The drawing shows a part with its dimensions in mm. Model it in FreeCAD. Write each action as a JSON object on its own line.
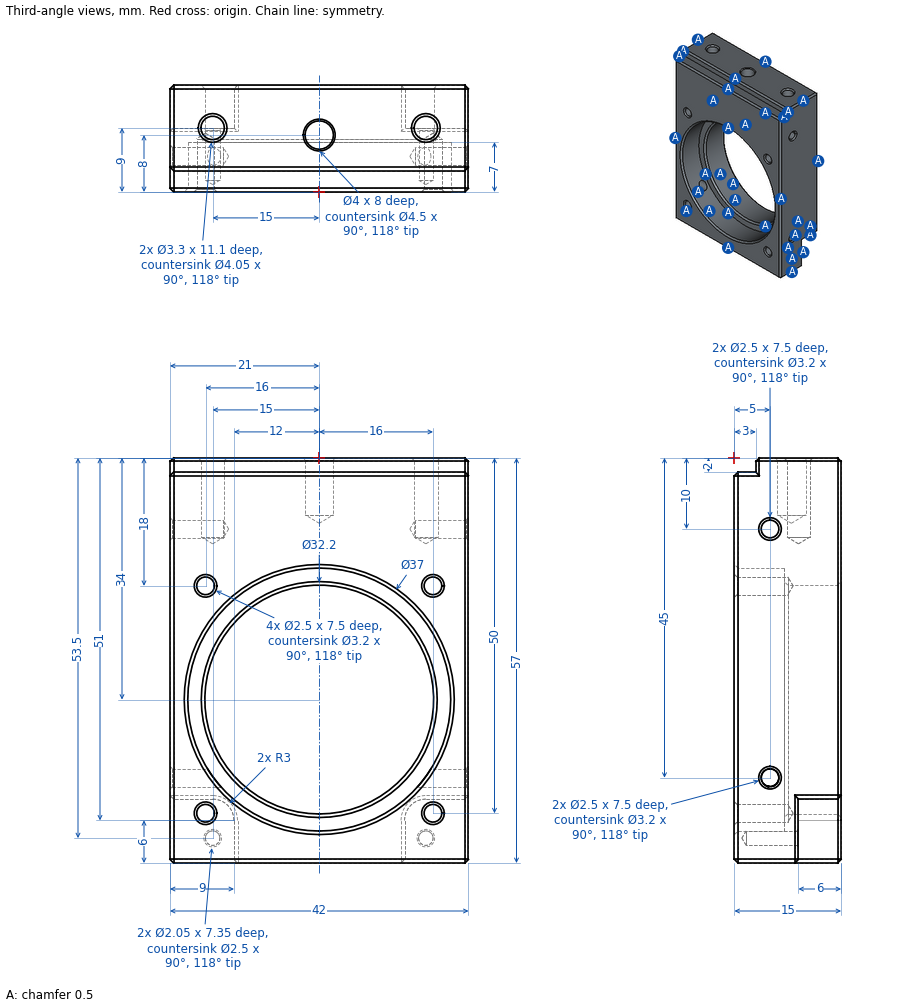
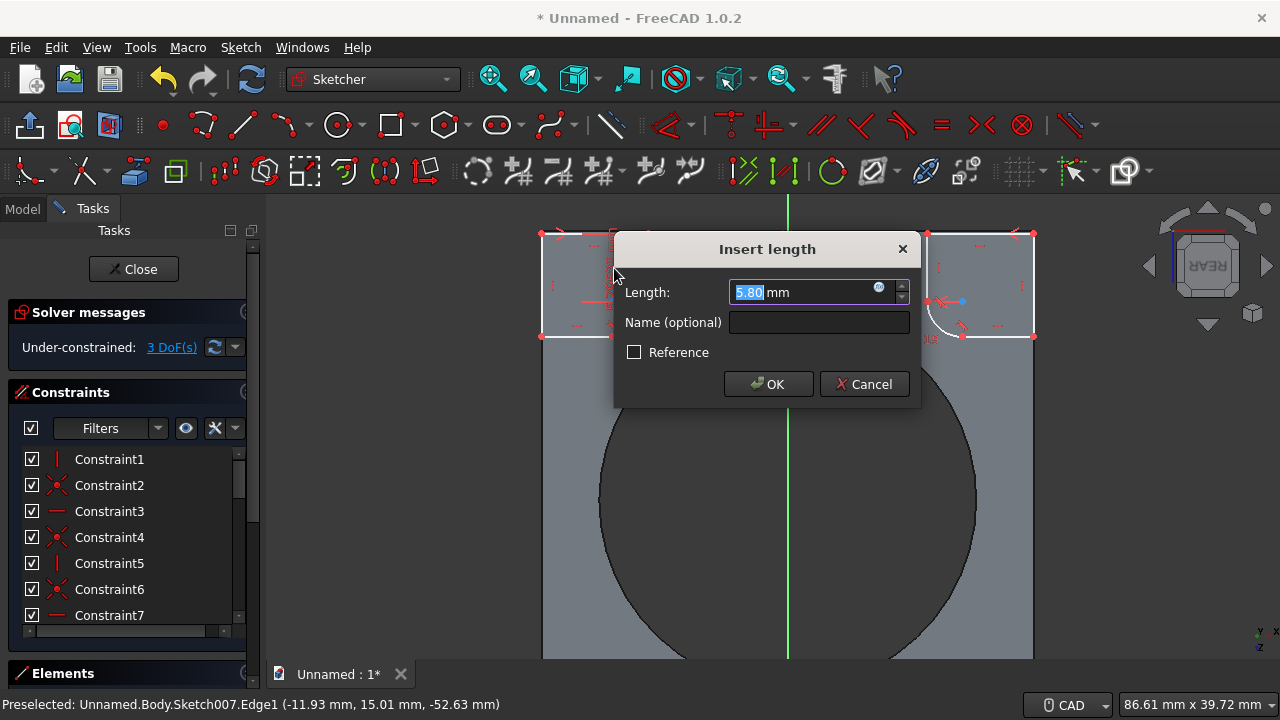
{"action": "type", "text": "6"}
{"action": "key", "text": "Return"}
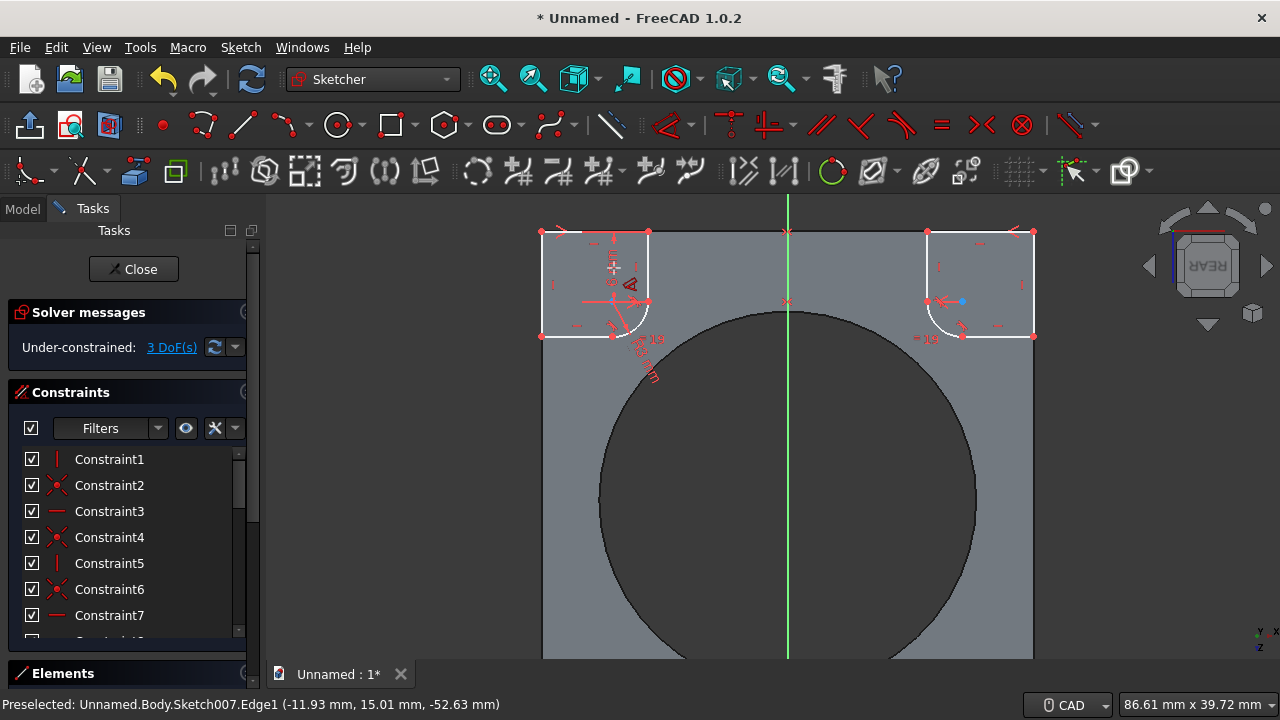
{"action": "left_click", "coordinate": [616, 232]}
{"action": "left_click", "coordinate": [595, 290]}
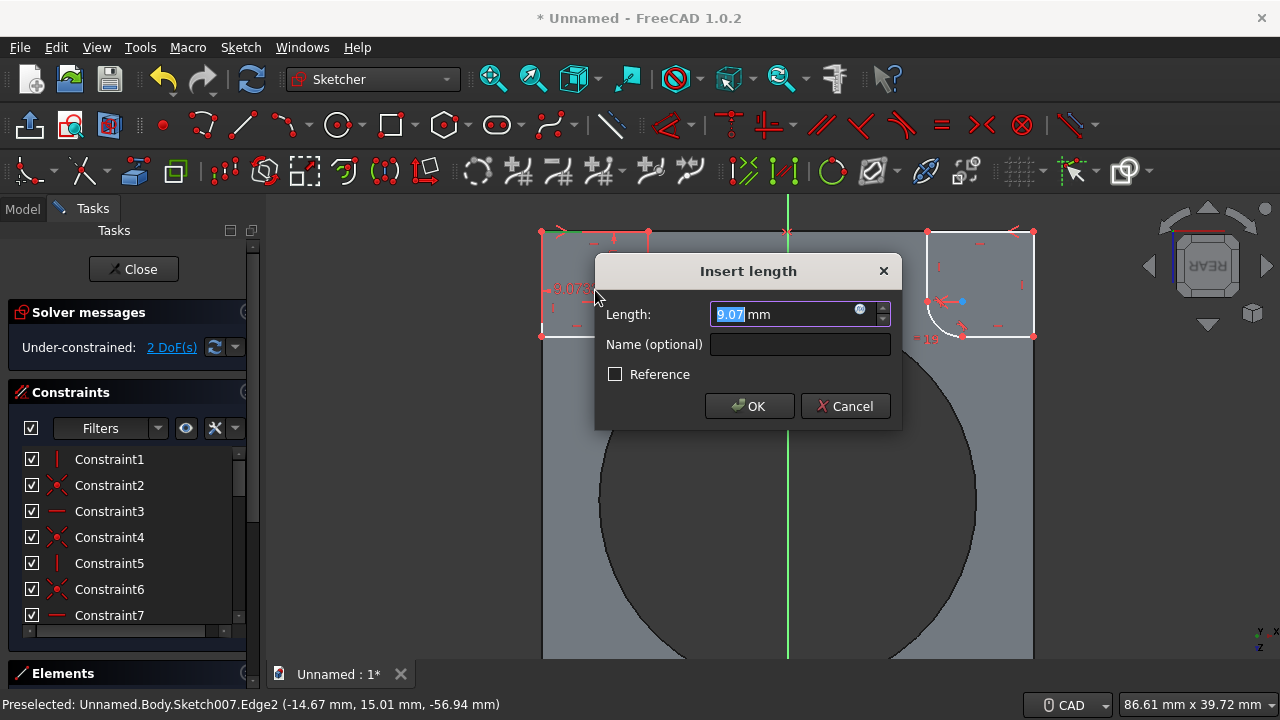
{"action": "type", "text": "9"}
{"action": "key", "text": "Return"}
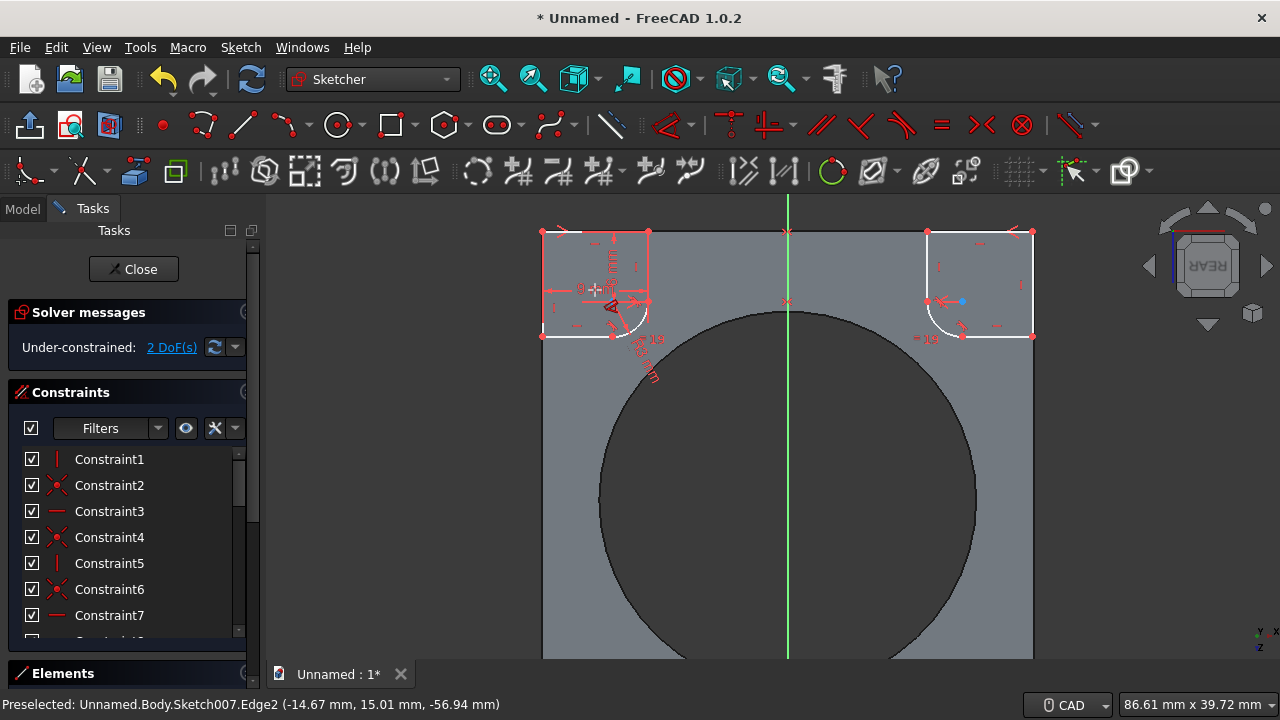
{"action": "left_click", "coordinate": [648, 302]}
{"action": "left_click", "coordinate": [718, 268]}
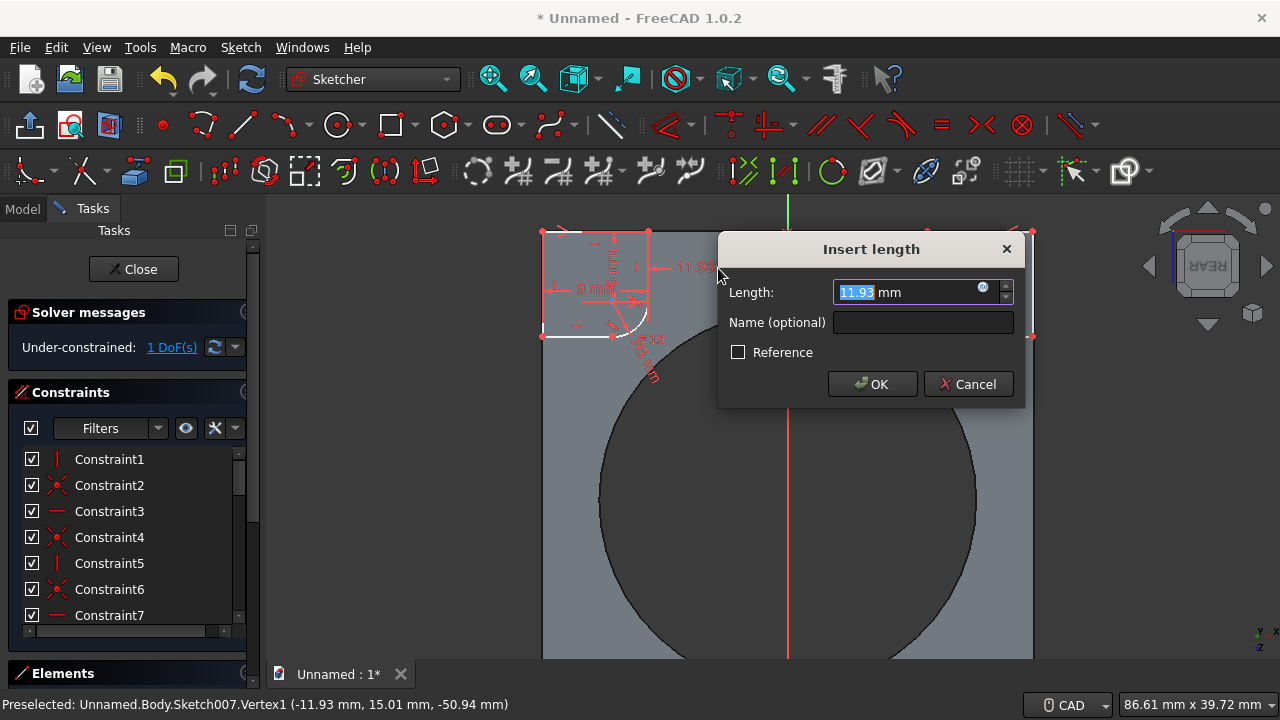
{"action": "type", "text": "12"}
{"action": "key", "text": "Return"}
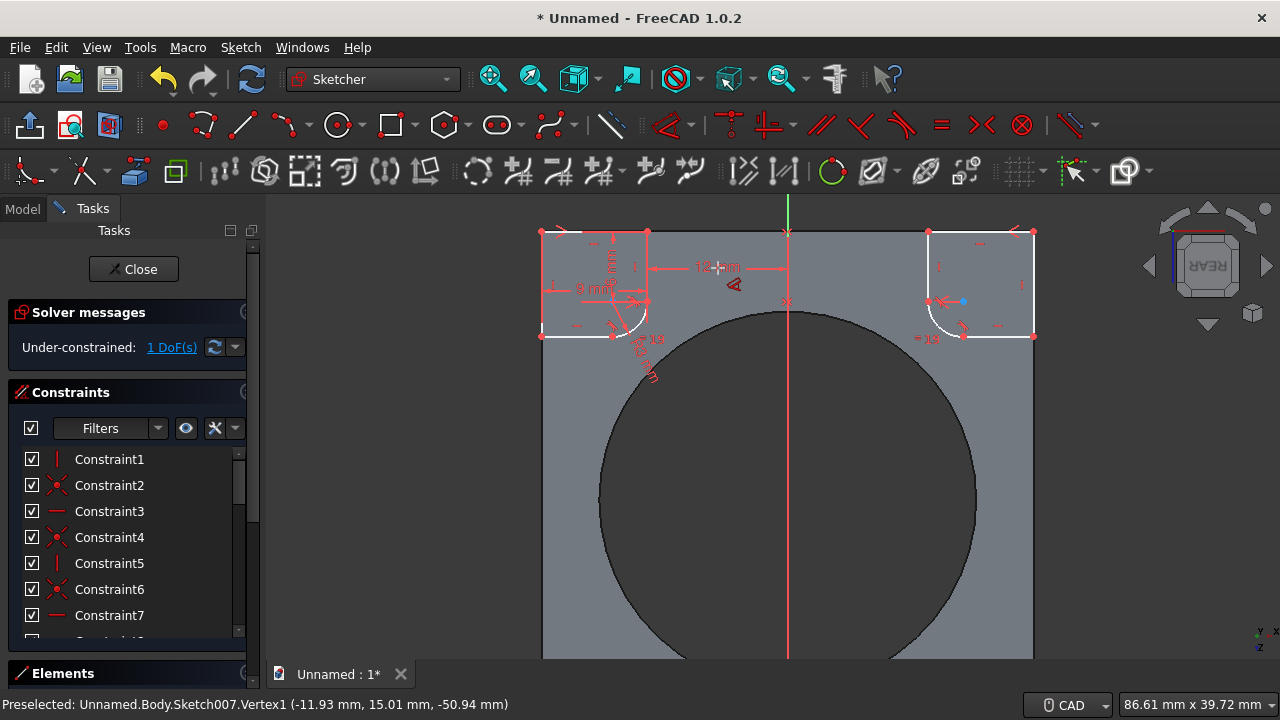
{"action": "left_click", "coordinate": [647, 302]}
{"action": "left_click", "coordinate": [613, 466]}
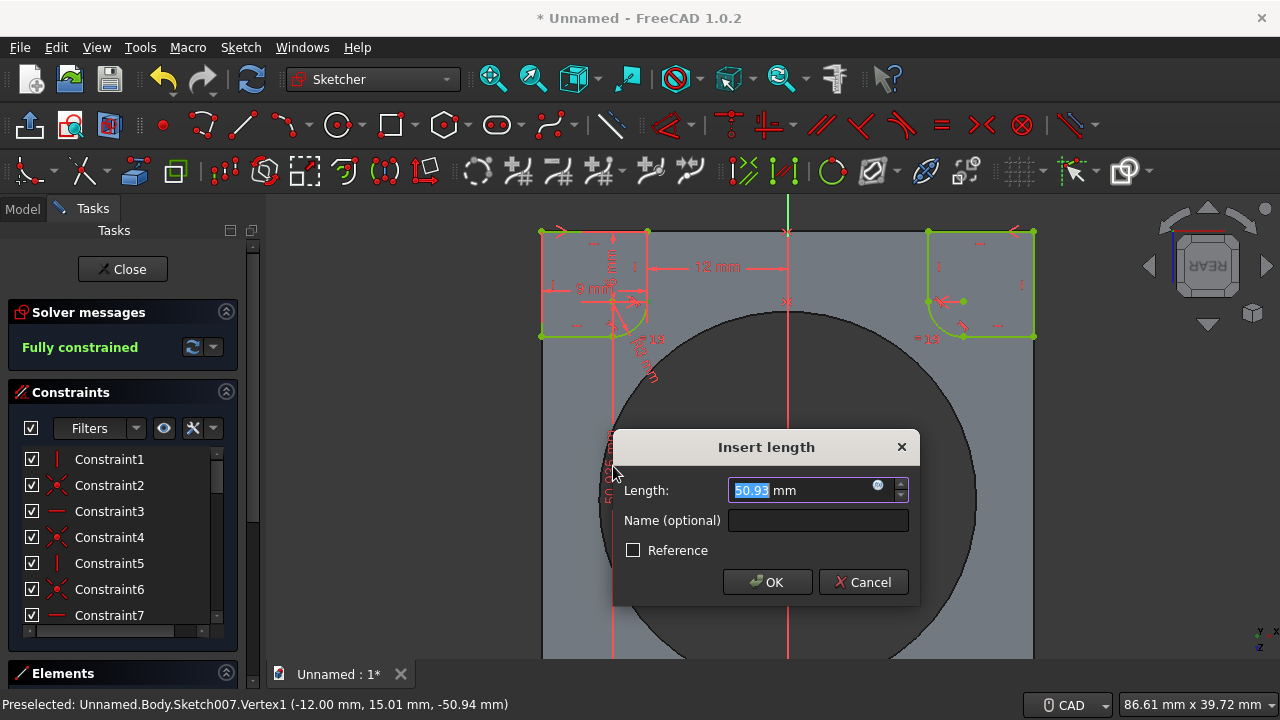
{"action": "type", "text": "51"}
{"action": "key", "text": "Return"}
{"action": "key", "text": "Escape"}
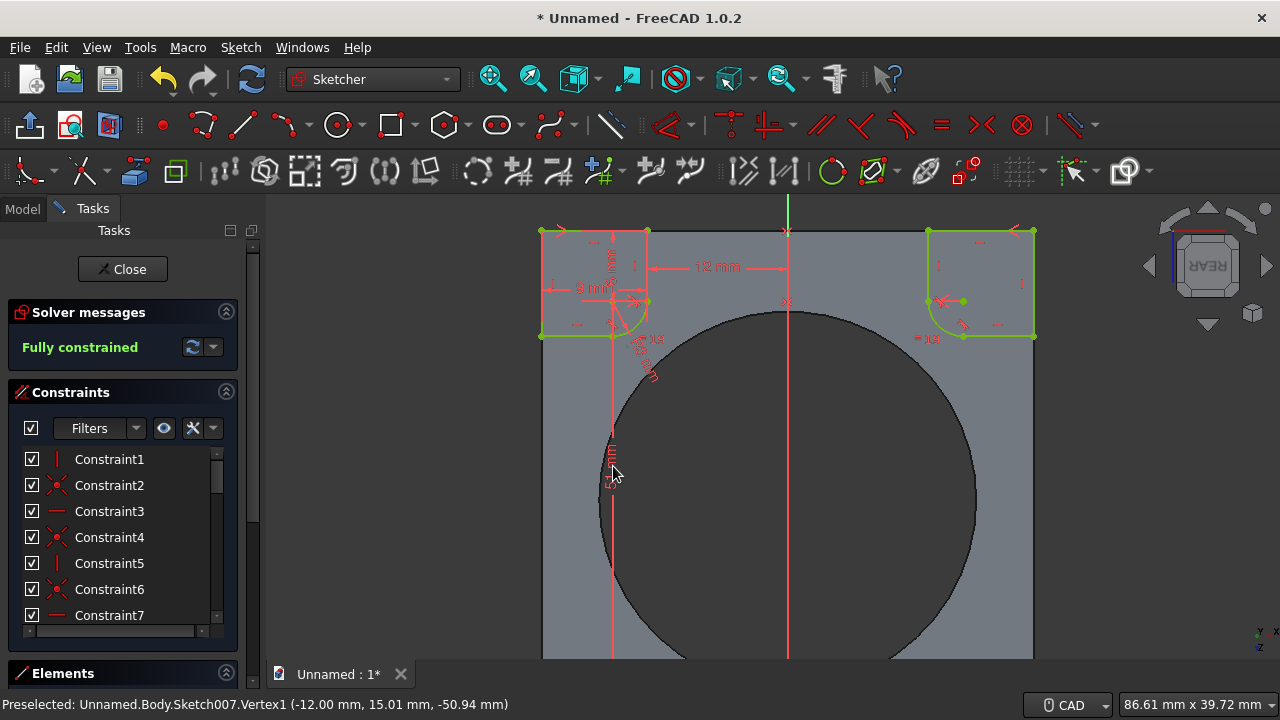
{"action": "left_click", "coordinate": [123, 269]}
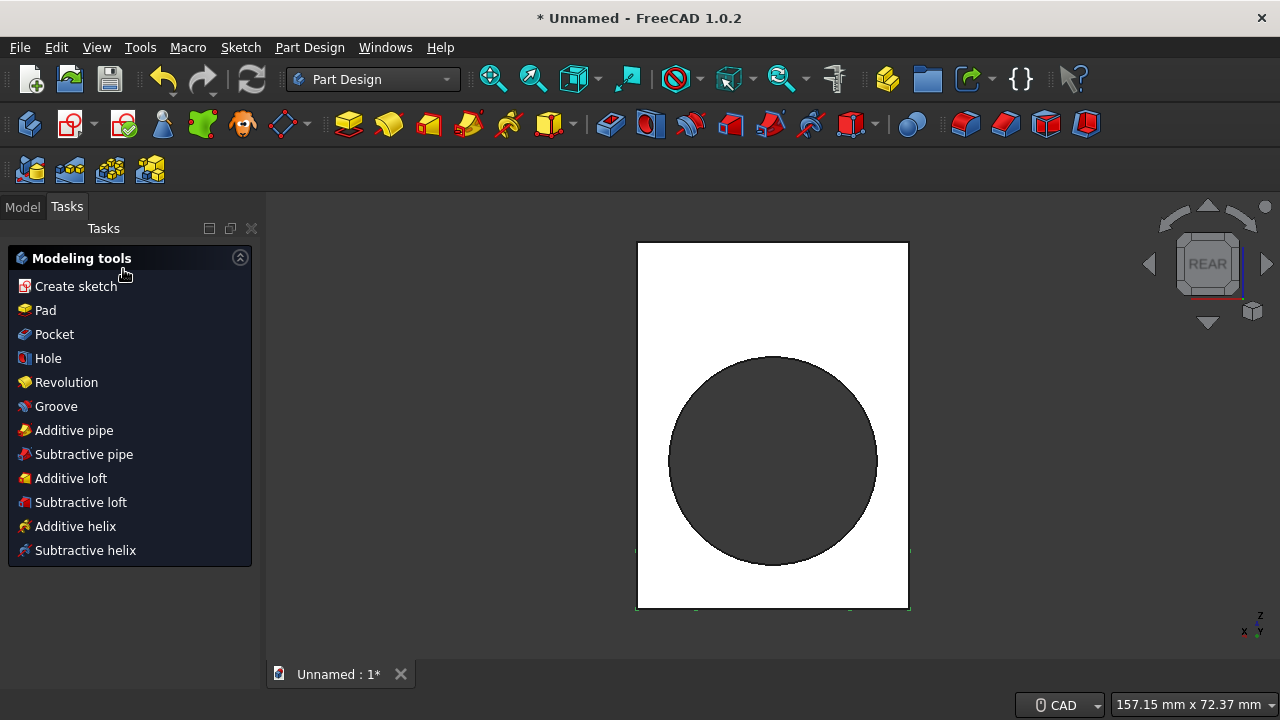
{"action": "left_click", "coordinate": [612, 124]}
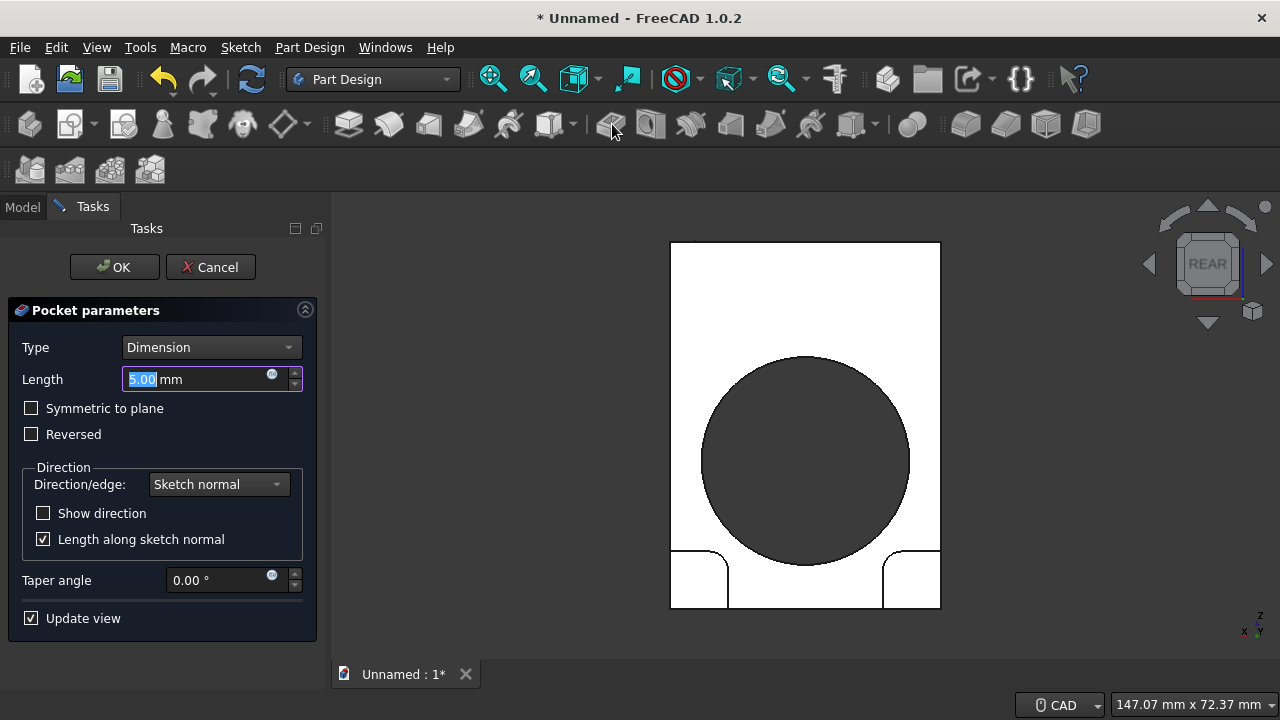
{"action": "type", "text": "6"}
{"action": "key", "text": "Tab"}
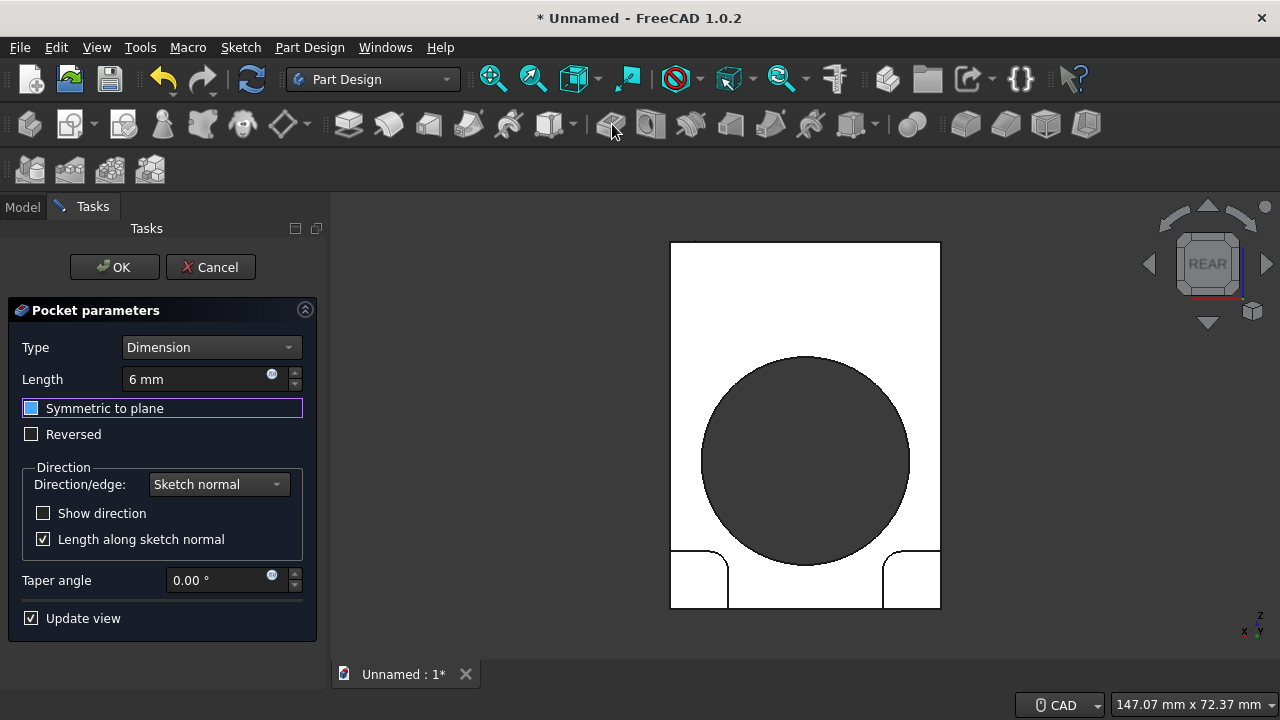
{"action": "left_click", "coordinate": [115, 267]}